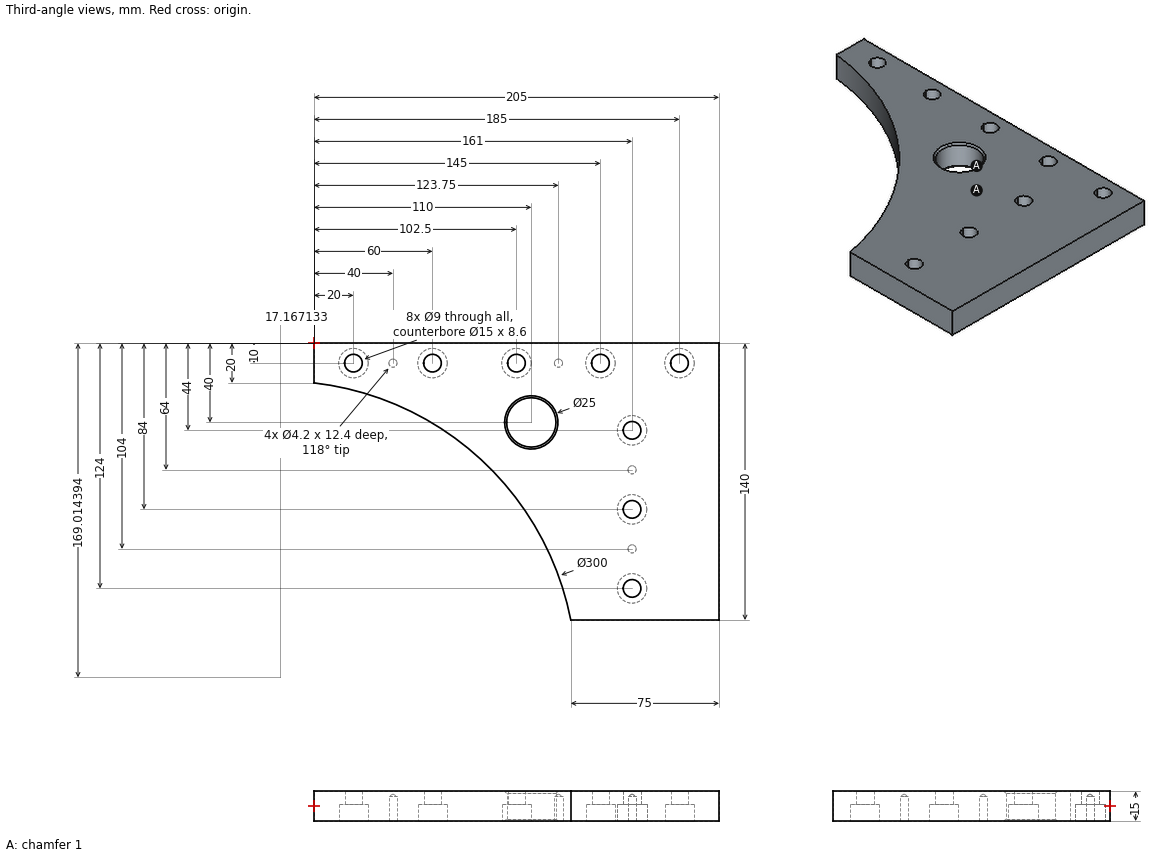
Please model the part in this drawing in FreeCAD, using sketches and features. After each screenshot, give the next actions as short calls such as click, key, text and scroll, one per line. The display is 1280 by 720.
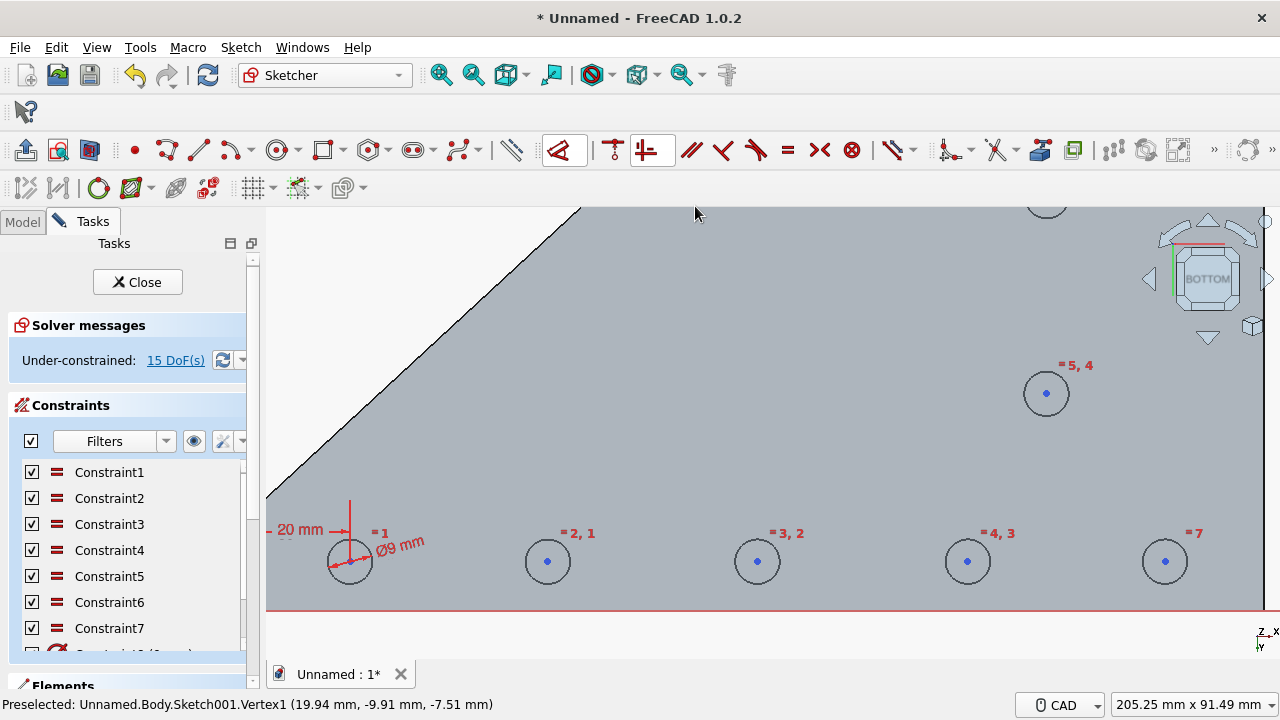
click(350, 562)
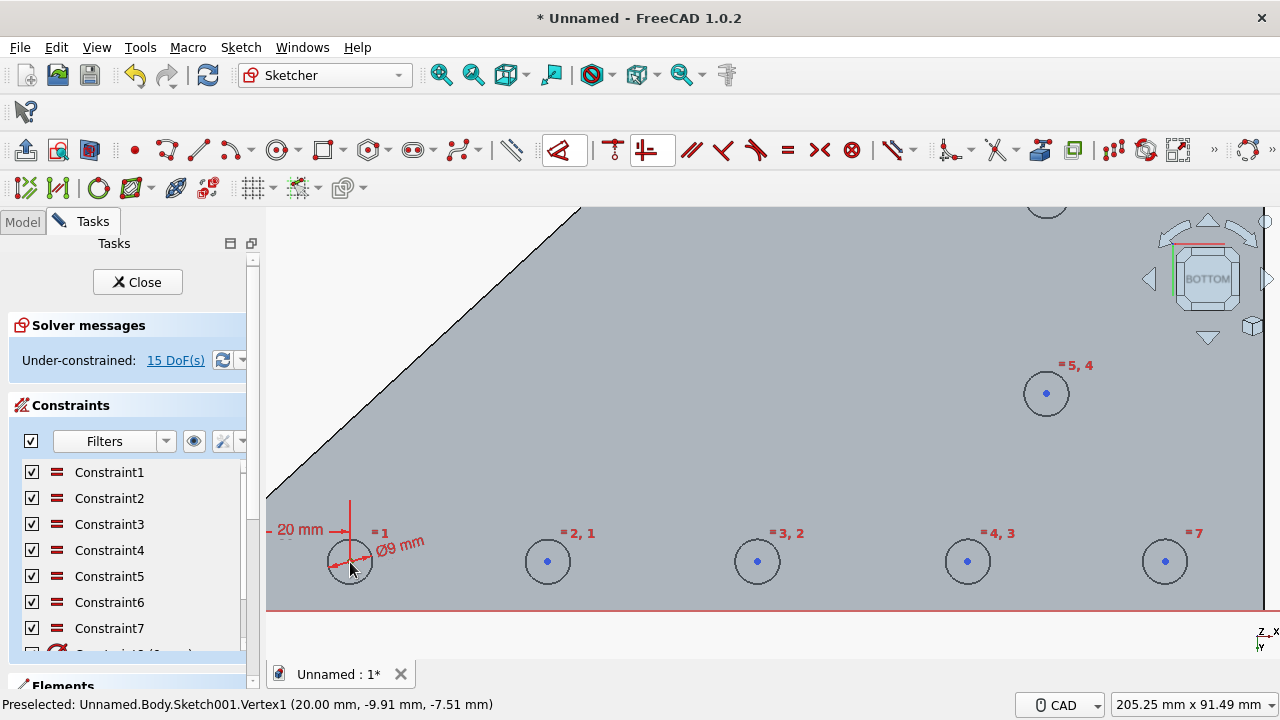
click(582, 150)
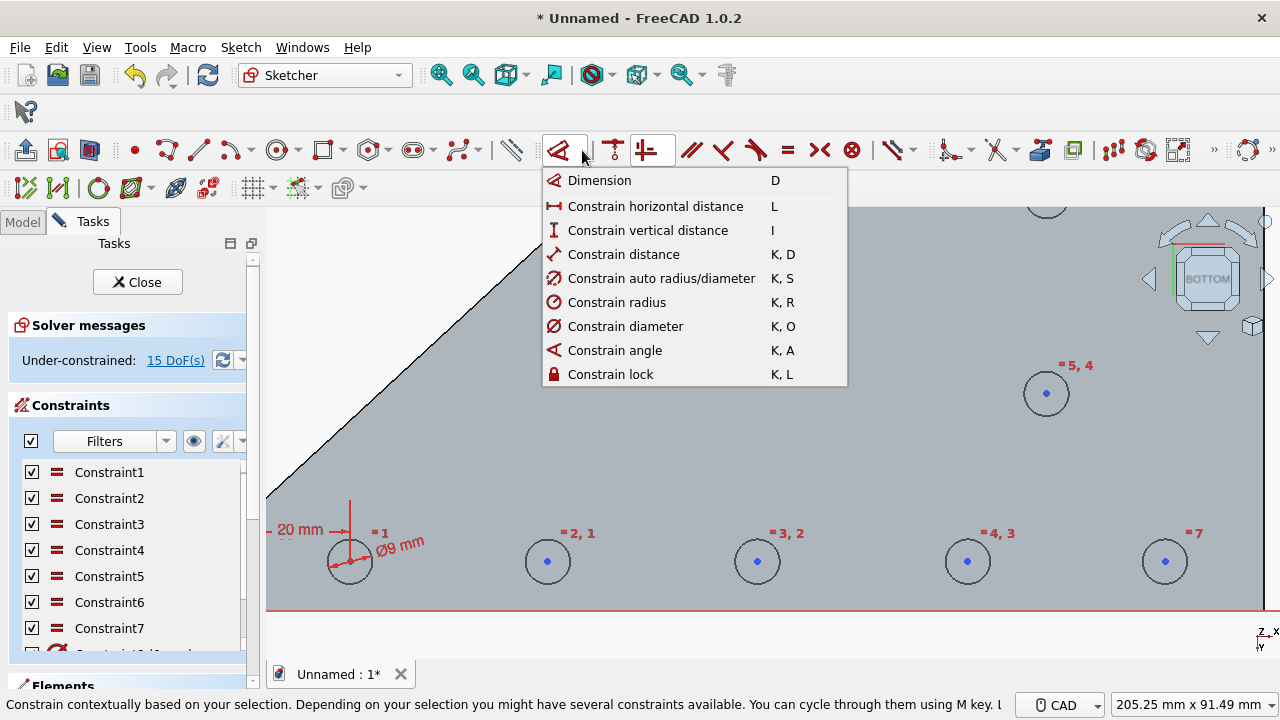
click(695, 230)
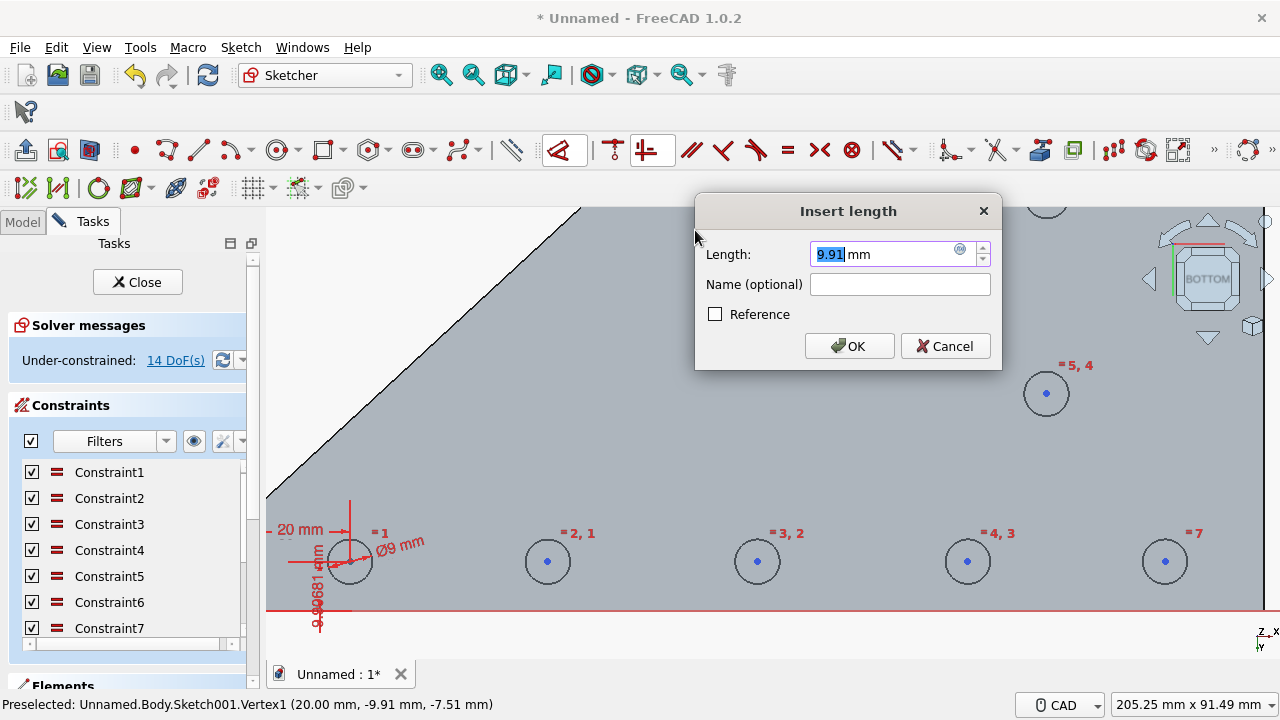
text(10)
key(Return)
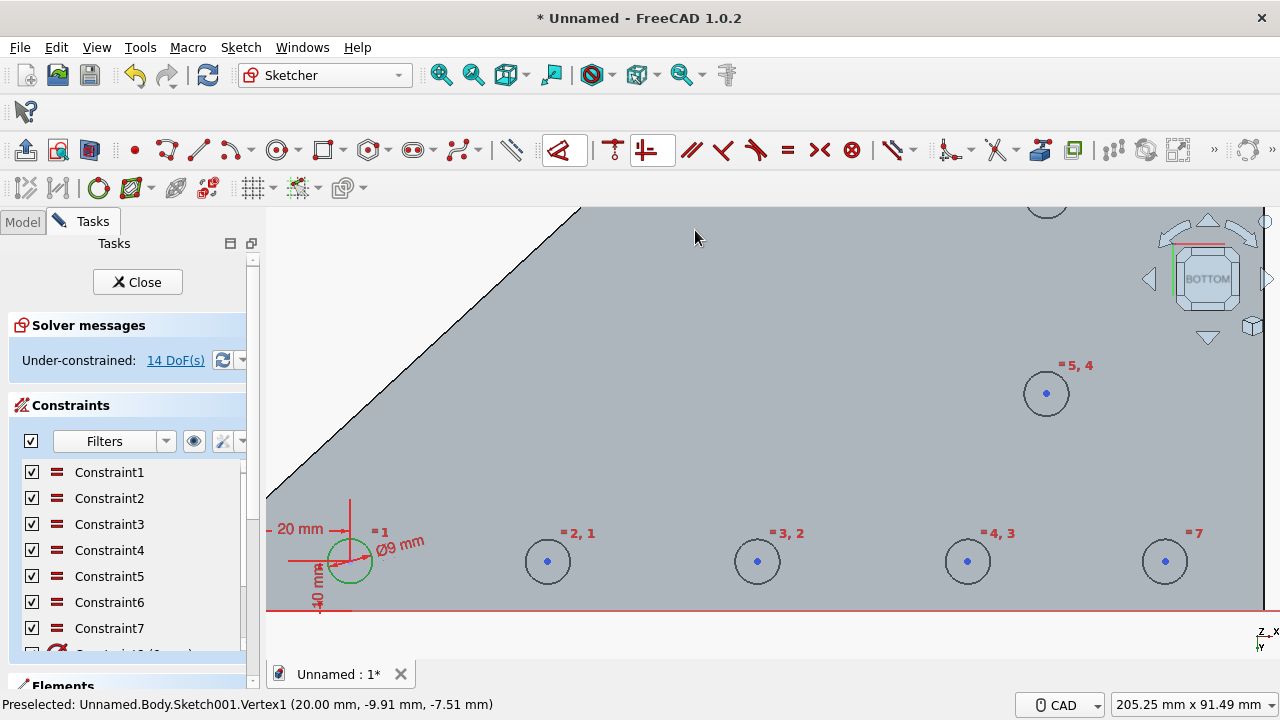
click(548, 562)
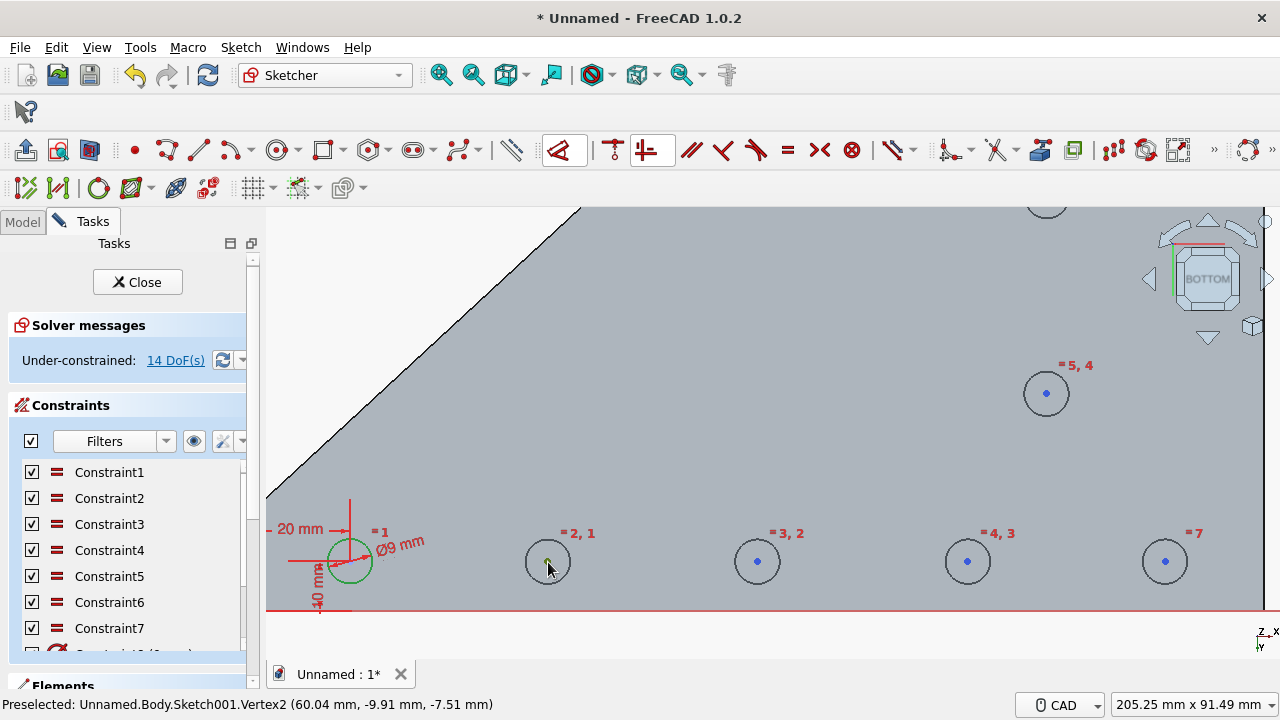
click(582, 150)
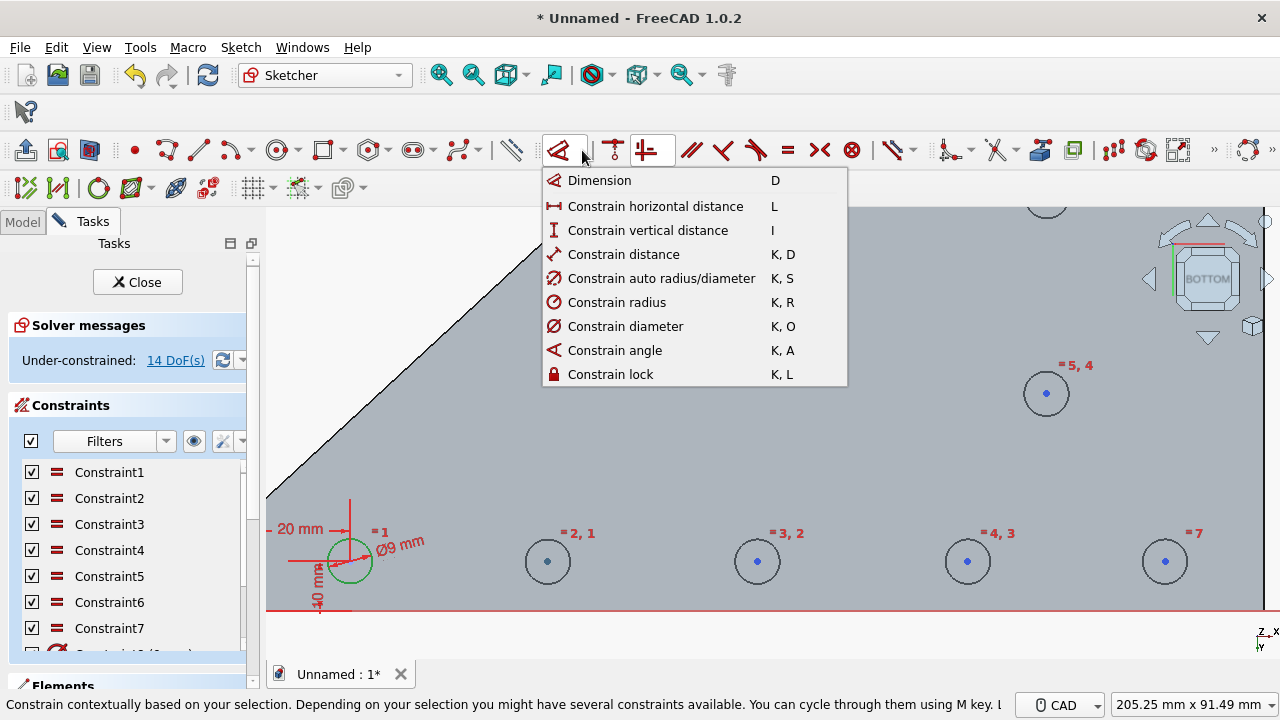
click(695, 206)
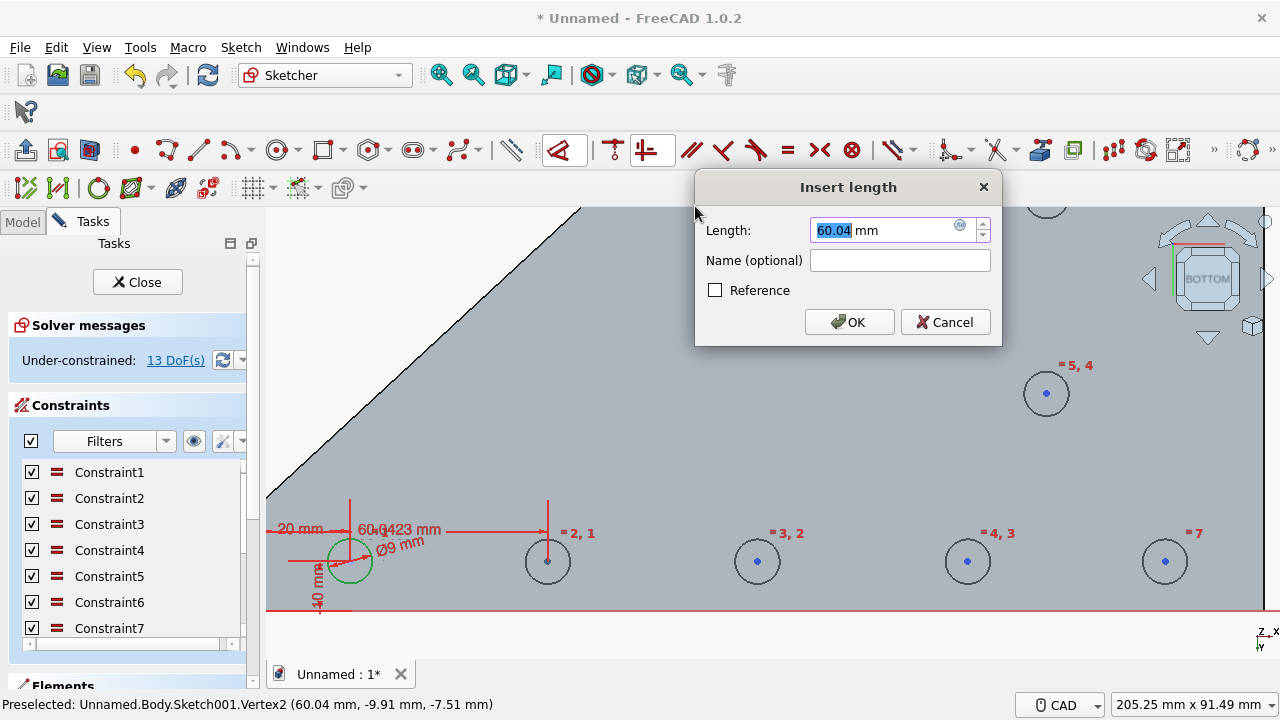
text(60)
key(Return)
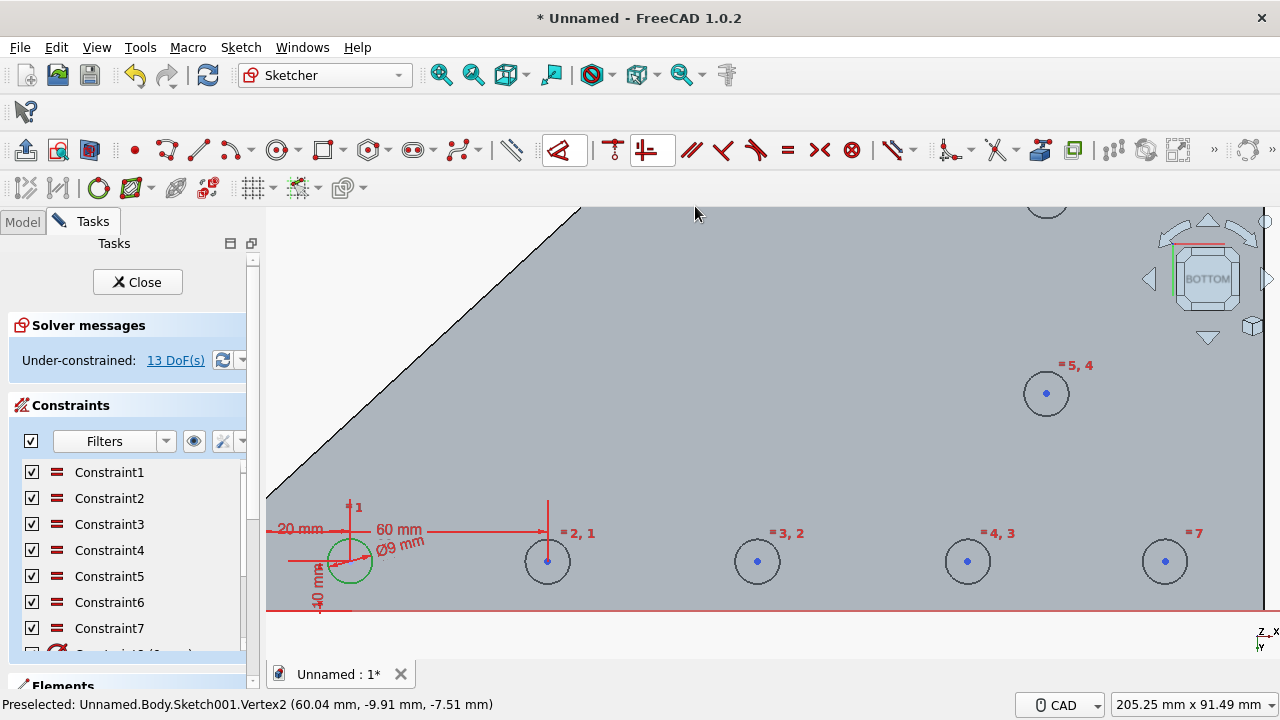
click(548, 562)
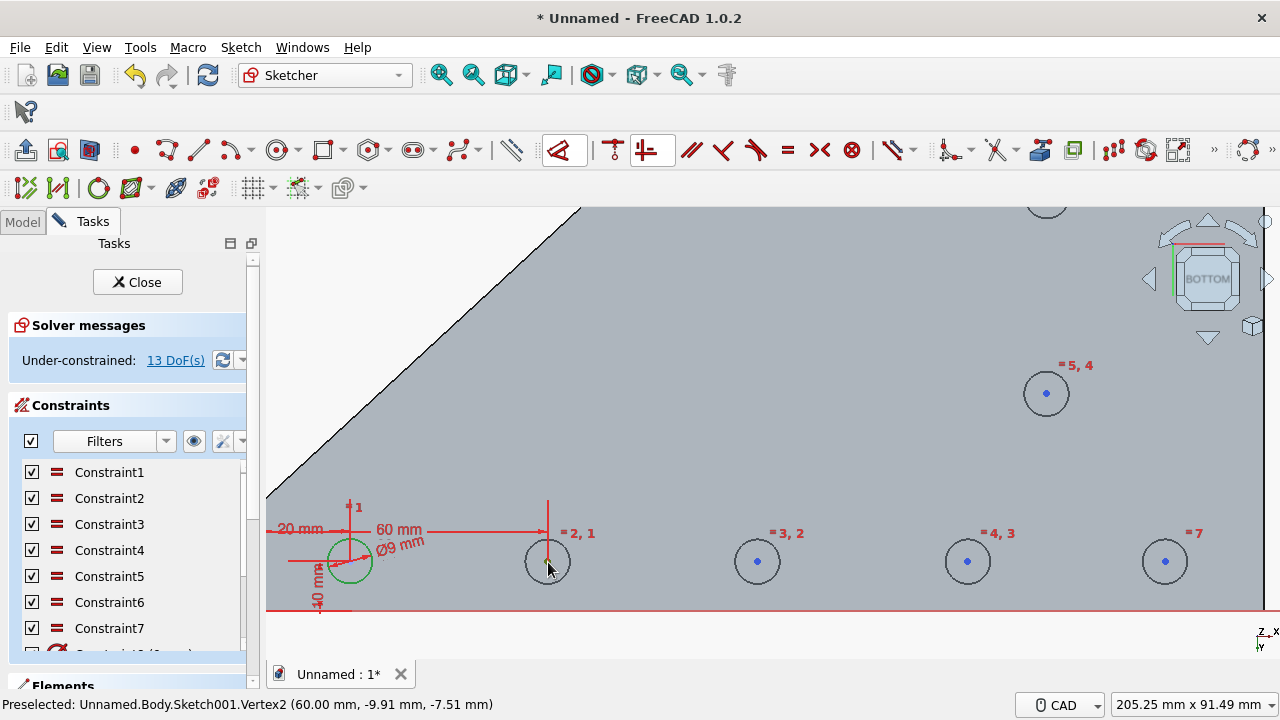
click(582, 150)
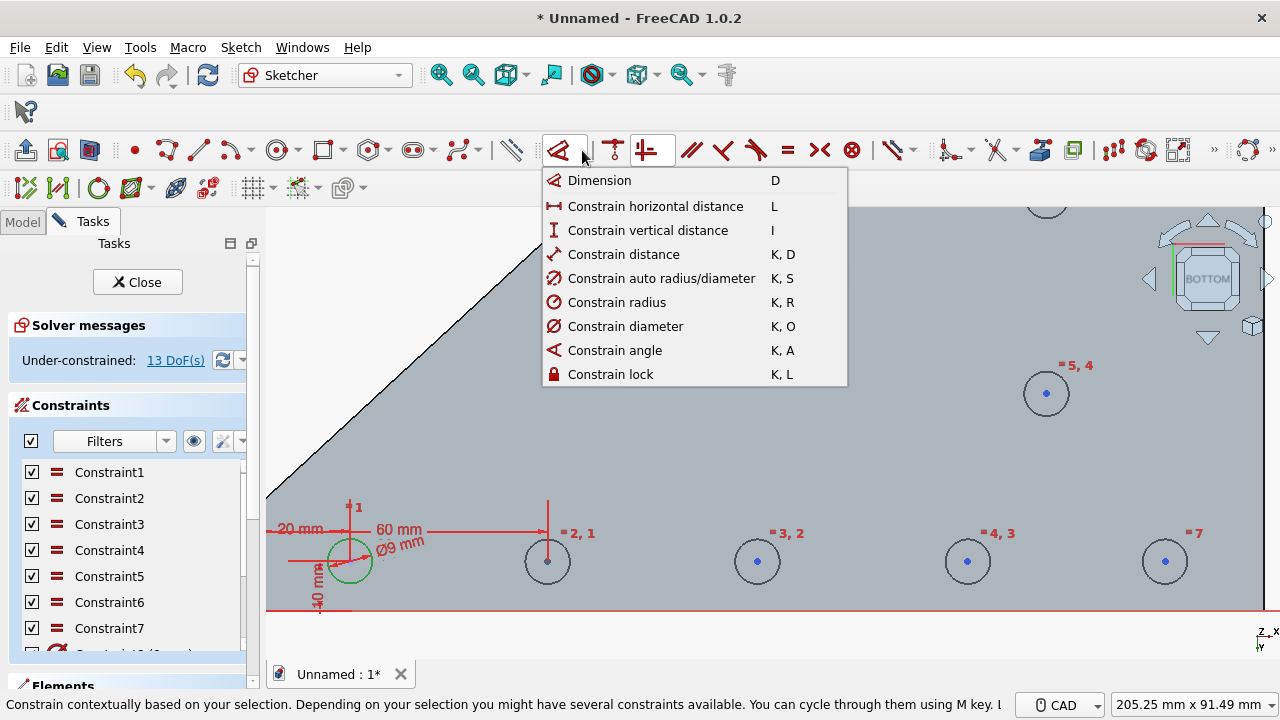
click(695, 230)